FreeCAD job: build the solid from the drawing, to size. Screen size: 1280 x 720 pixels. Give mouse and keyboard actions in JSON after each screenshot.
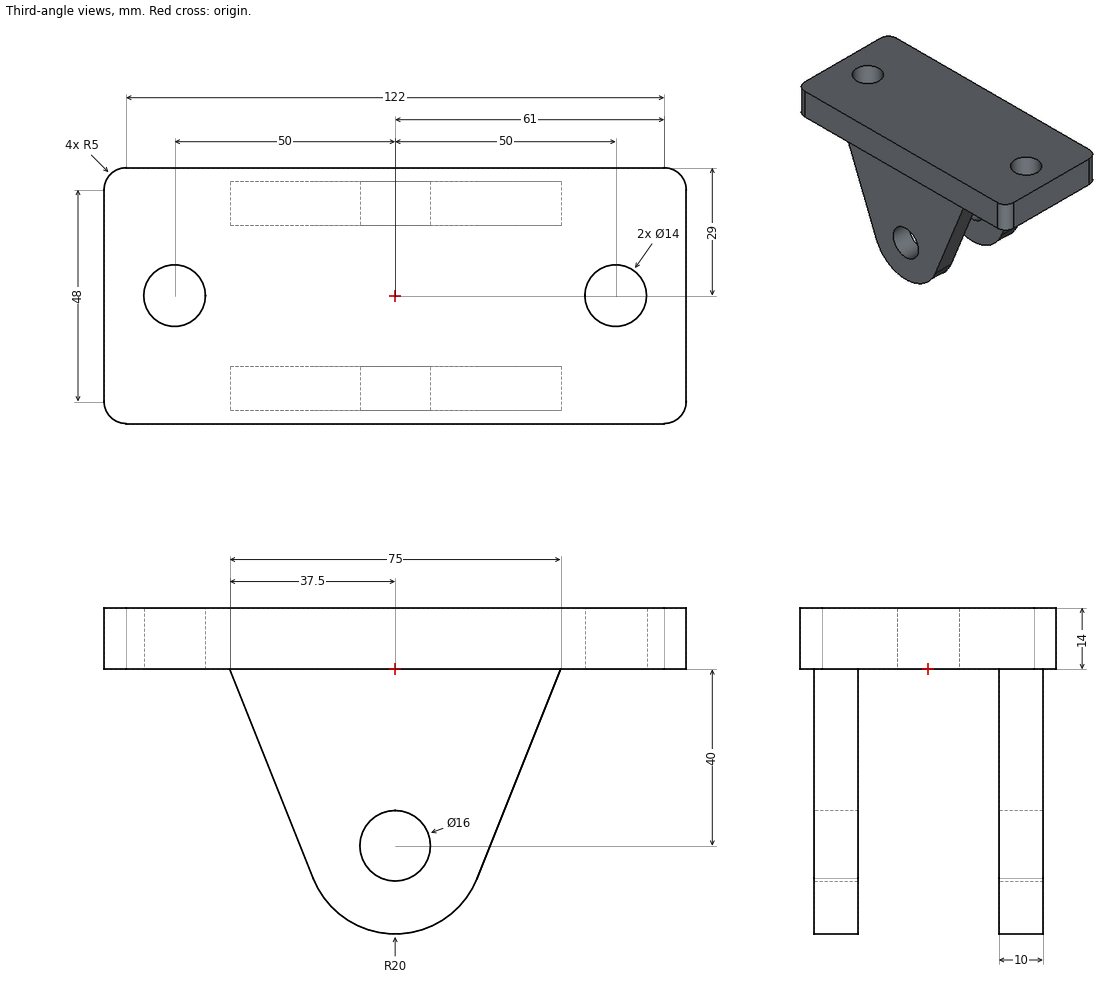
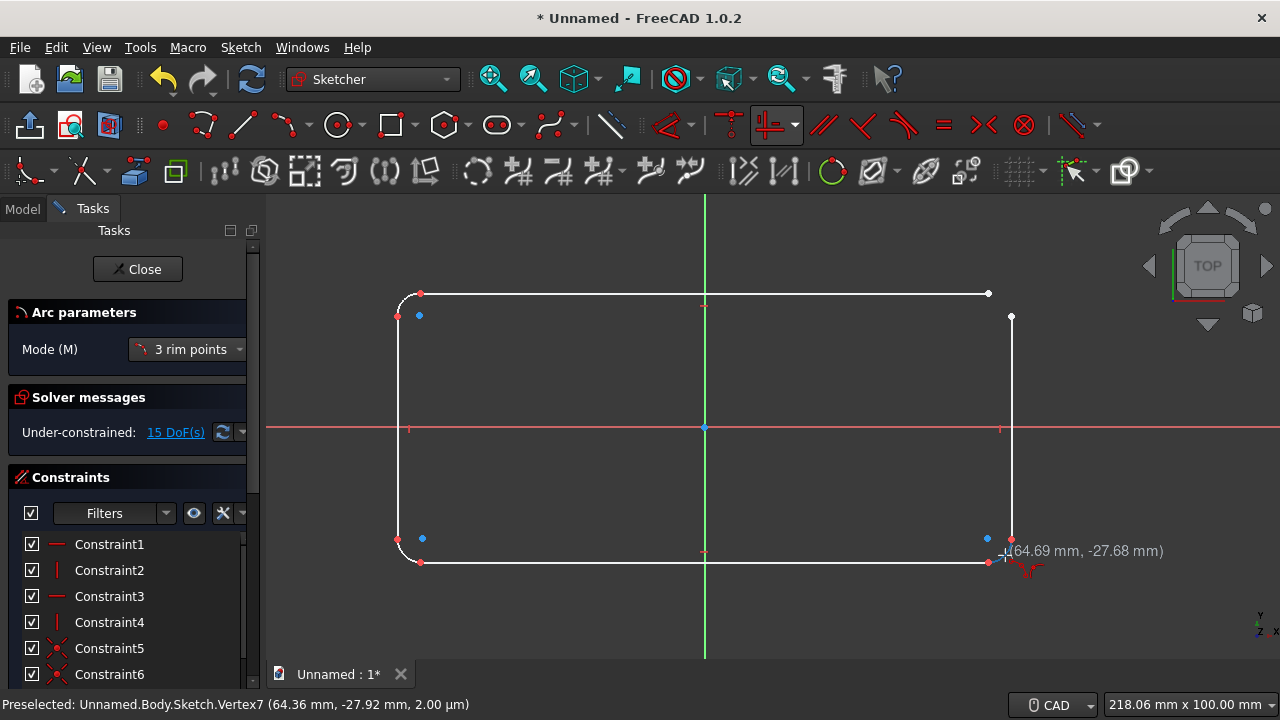
{"action": "left_click", "coordinate": [1012, 317]}
{"action": "left_click", "coordinate": [989, 294]}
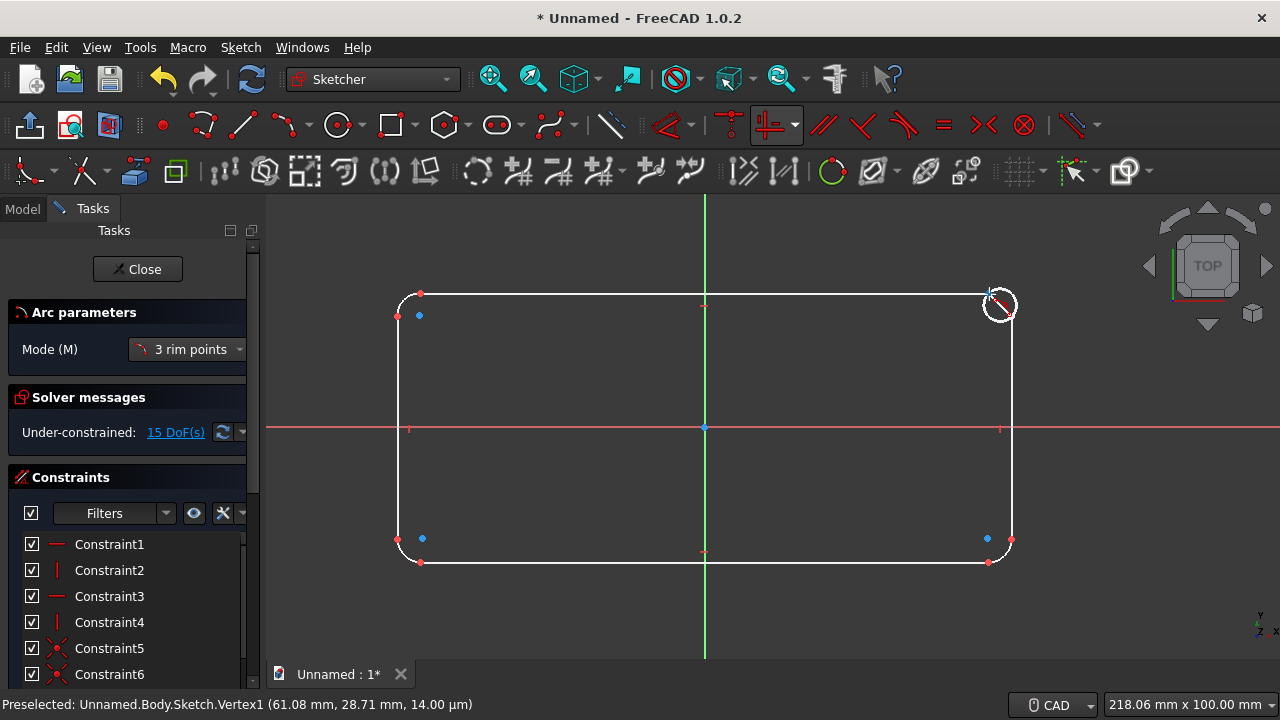
{"action": "scroll", "coordinate": [1005, 299], "scroll_direction": "up", "scroll_amount": 5}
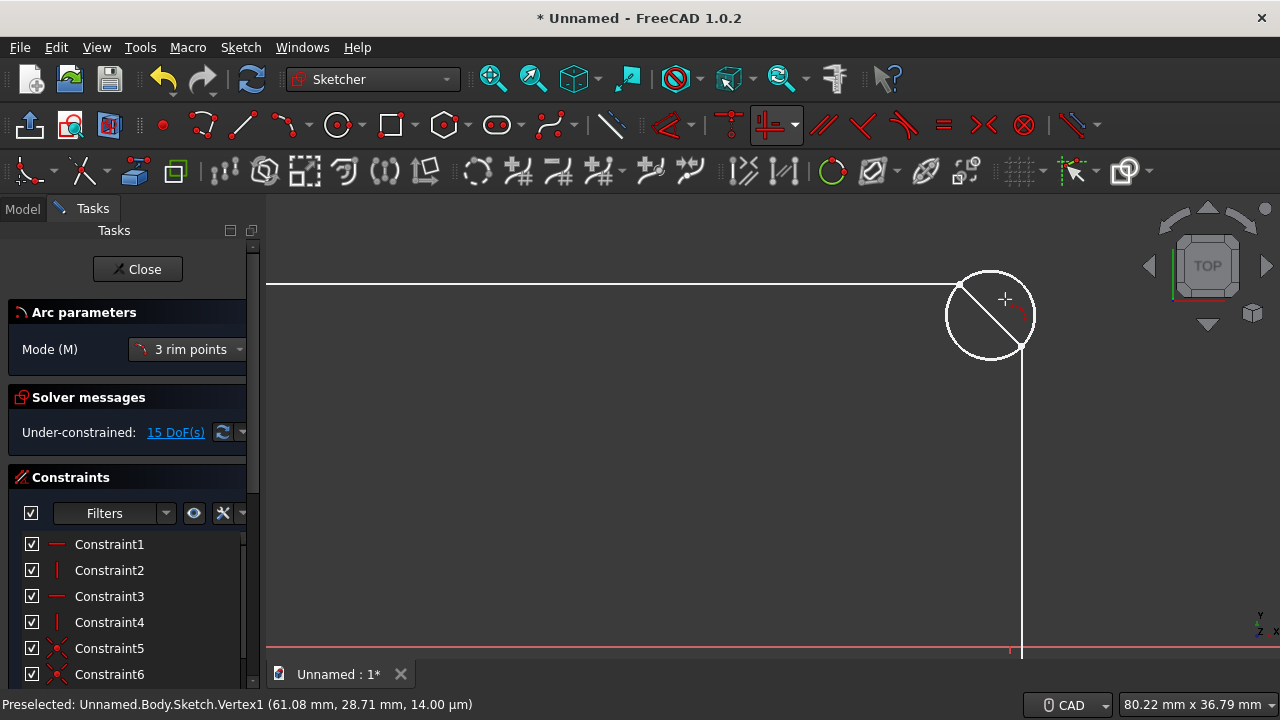
{"action": "left_click", "coordinate": [1003, 299]}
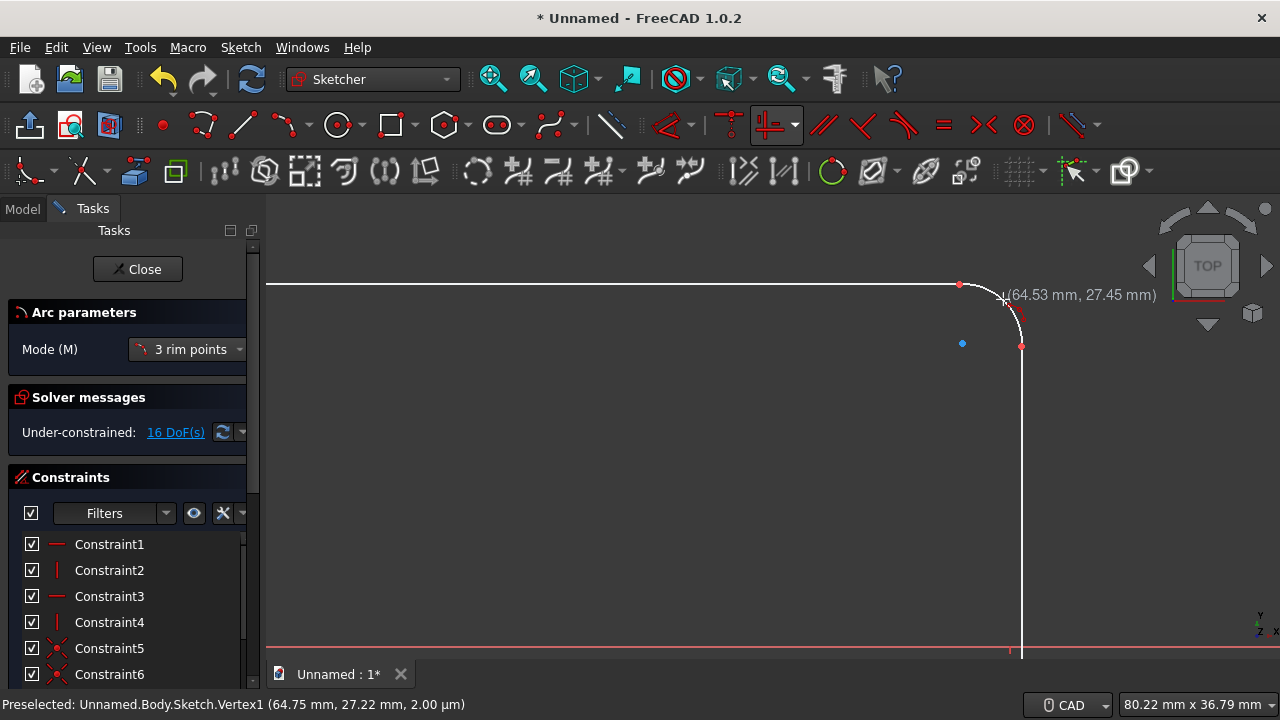
{"action": "left_click", "coordinate": [338, 126]}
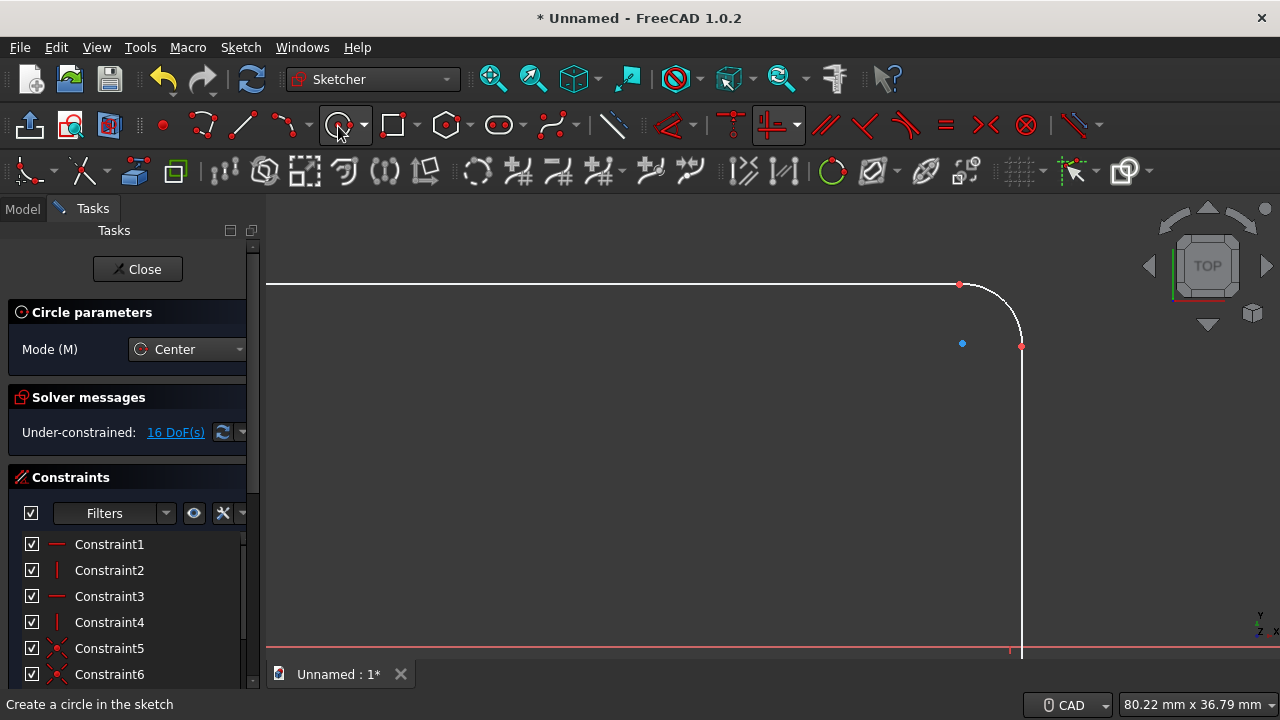
{"action": "scroll", "coordinate": [1005, 298], "scroll_direction": "down", "scroll_amount": 5}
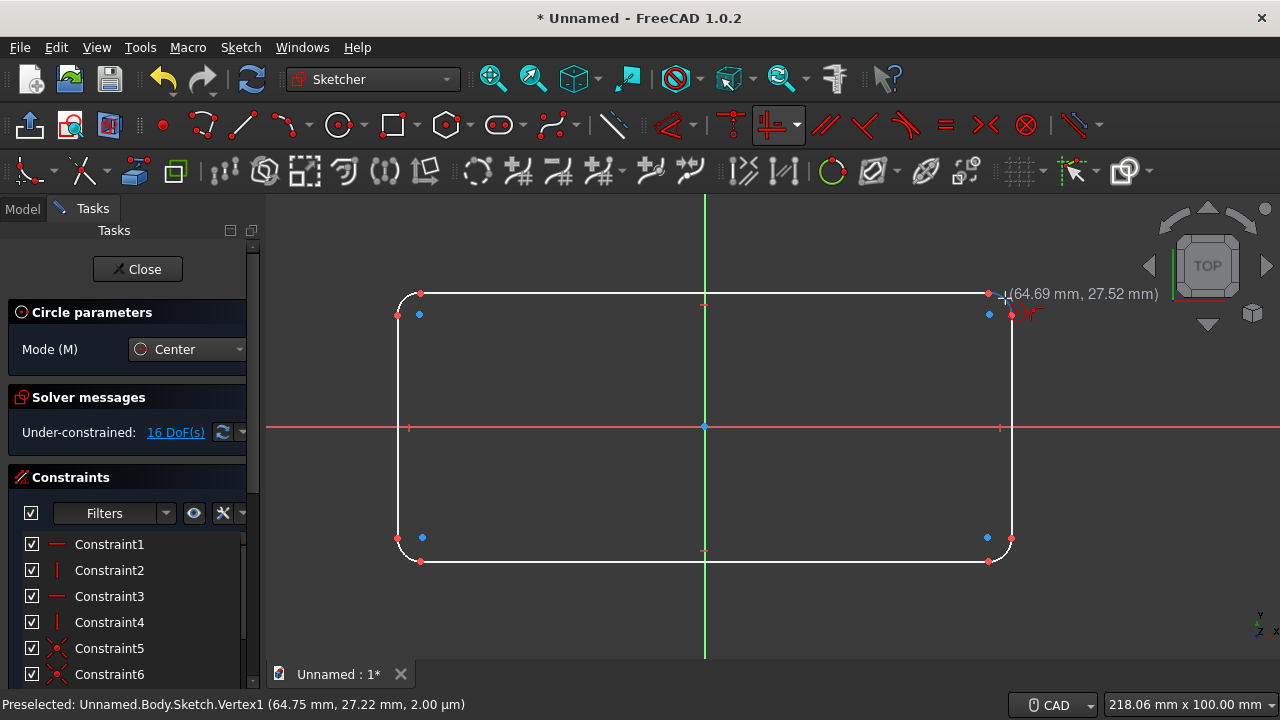
{"action": "left_click", "coordinate": [937, 427]}
{"action": "mouse_move", "coordinate": [960, 403]}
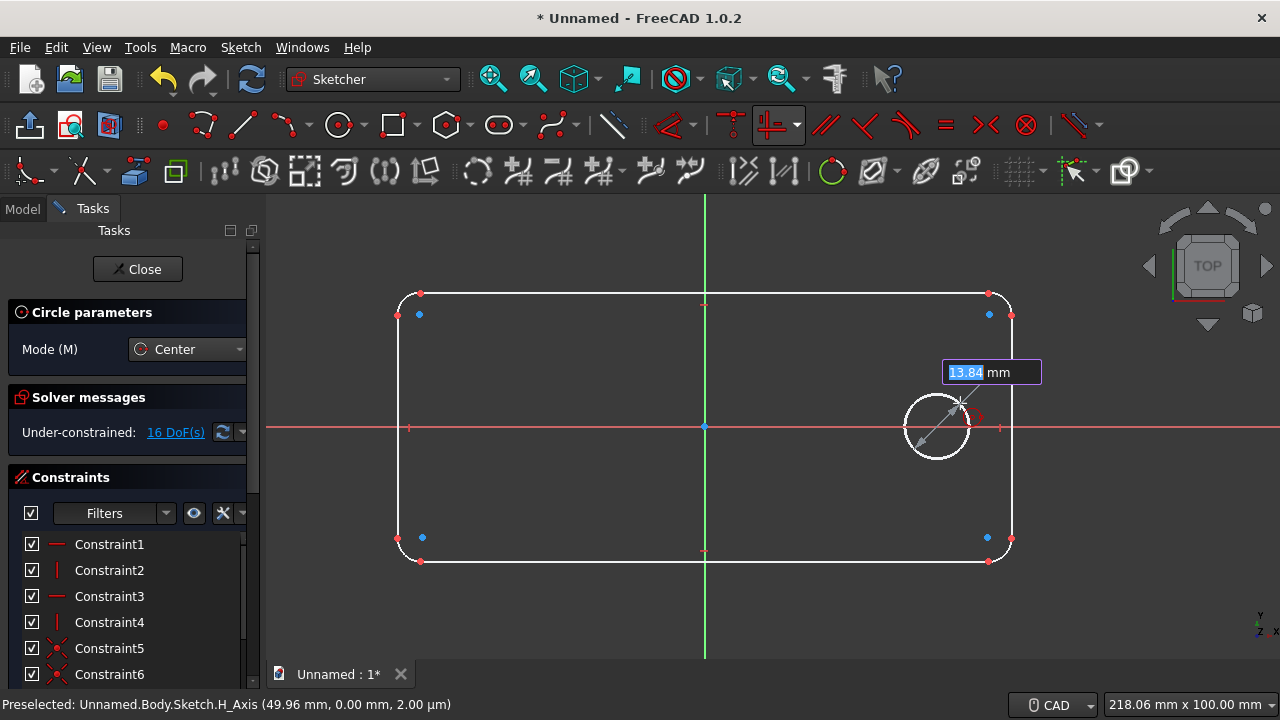
{"action": "type", "text": "14"}
{"action": "key", "text": "Return"}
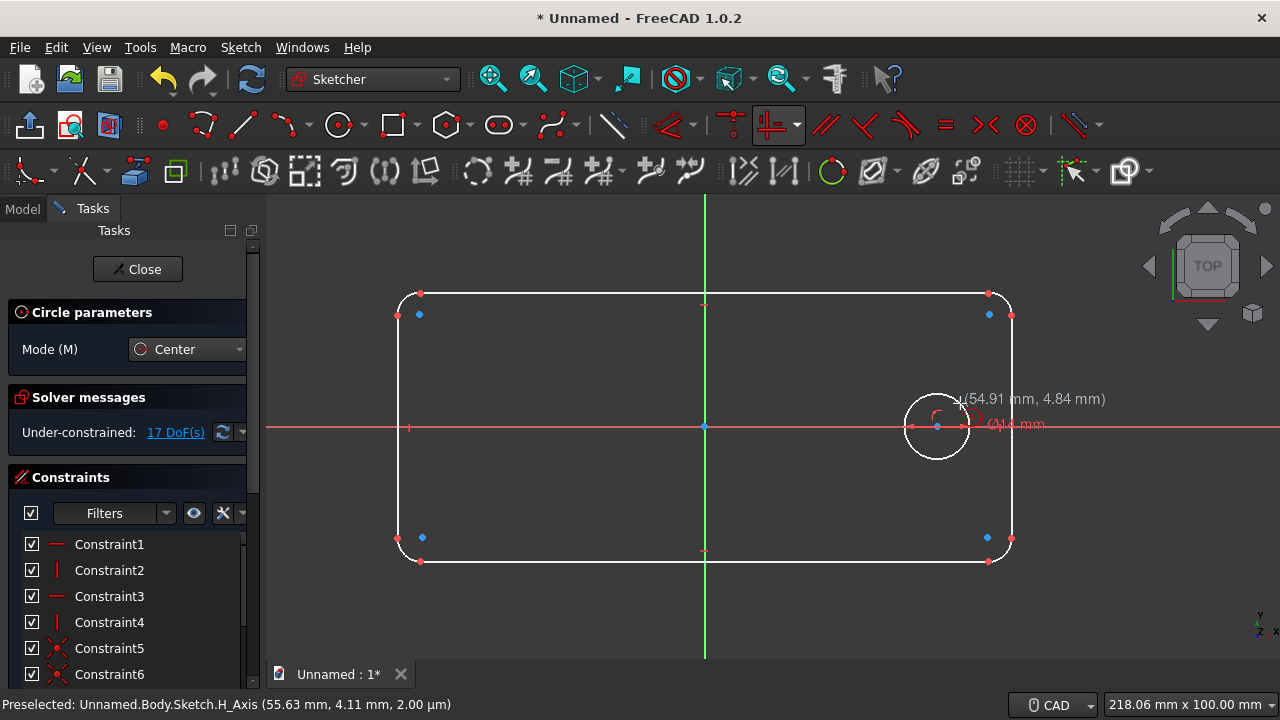
{"action": "left_click", "coordinate": [472, 427]}
{"action": "mouse_move", "coordinate": [495, 403]}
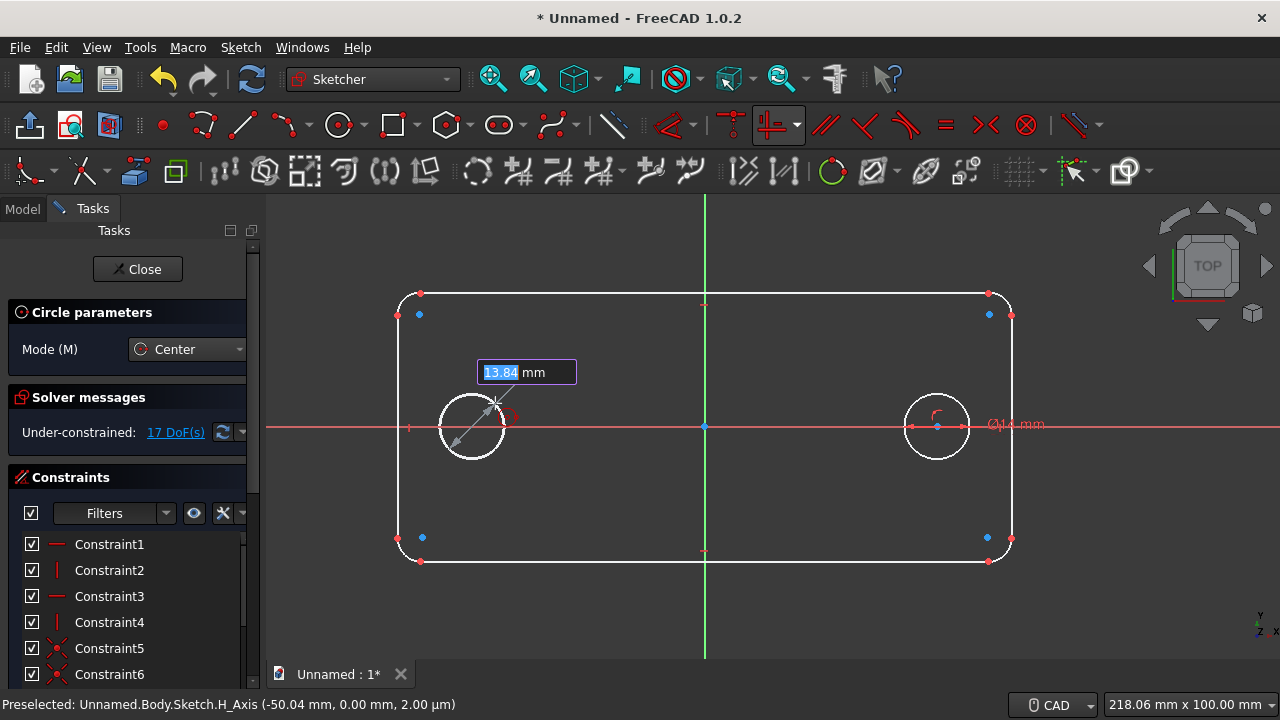
{"action": "type", "text": "14"}
{"action": "key", "text": "Return"}
{"action": "key", "text": "Escape"}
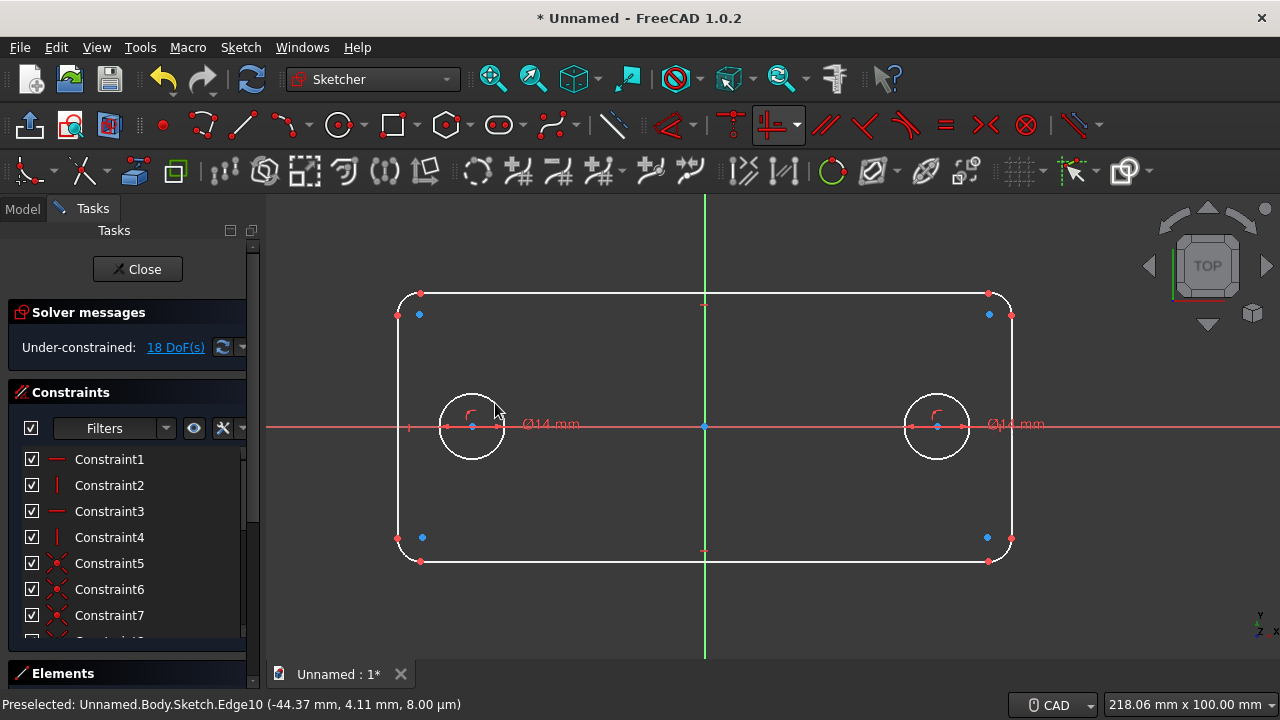
{"action": "left_click", "coordinate": [818, 293]}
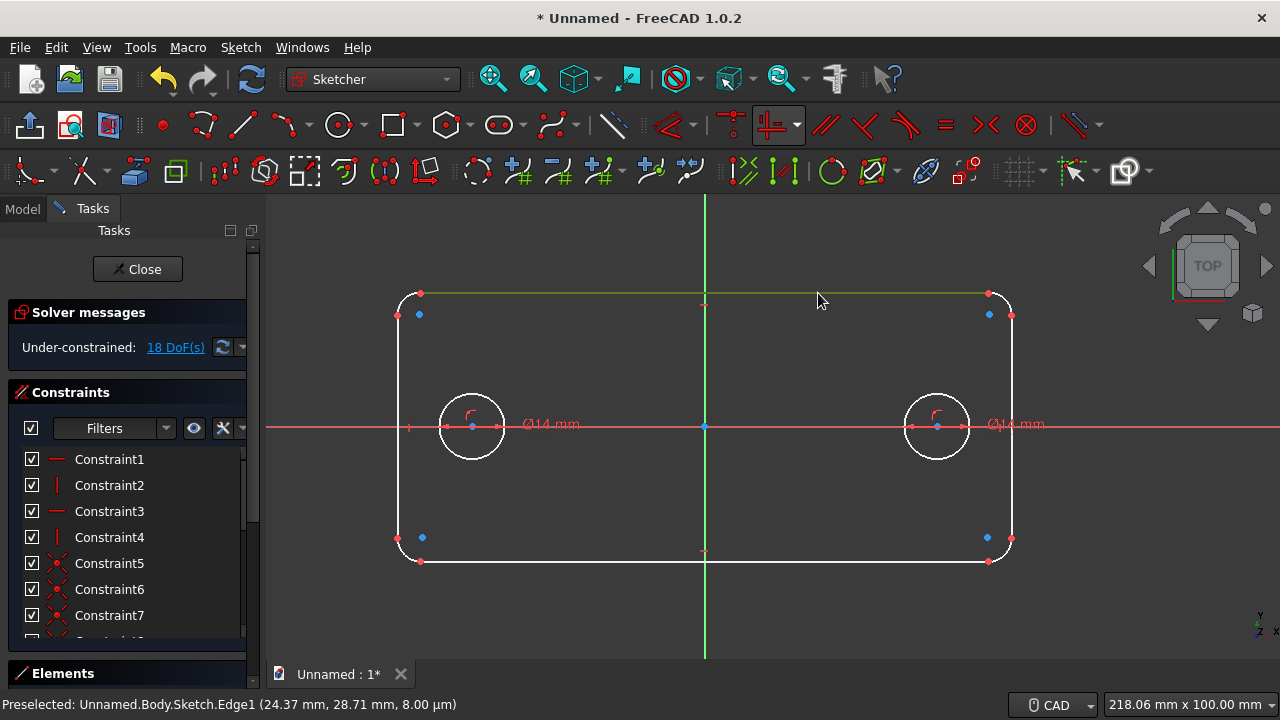
{"action": "scroll", "coordinate": [410, 295], "scroll_direction": "up", "scroll_amount": 2}